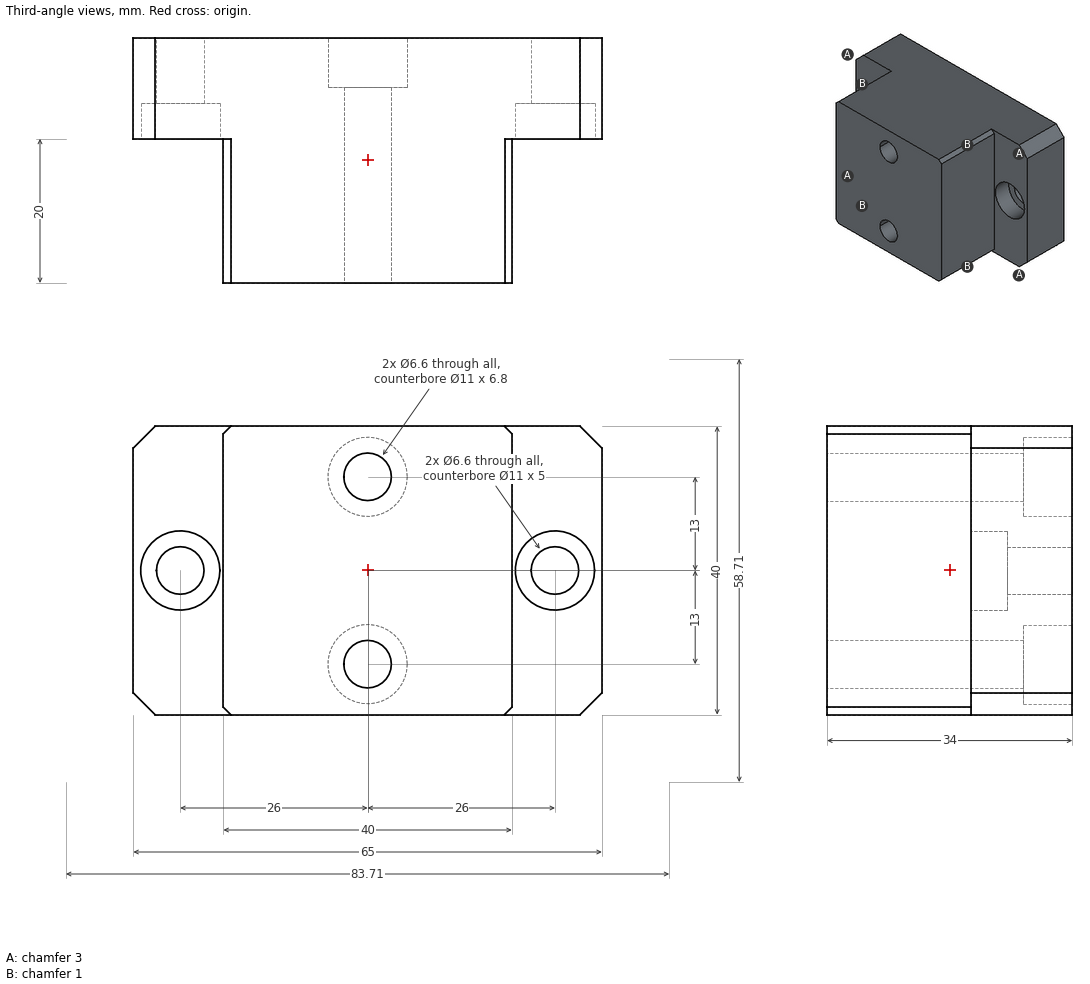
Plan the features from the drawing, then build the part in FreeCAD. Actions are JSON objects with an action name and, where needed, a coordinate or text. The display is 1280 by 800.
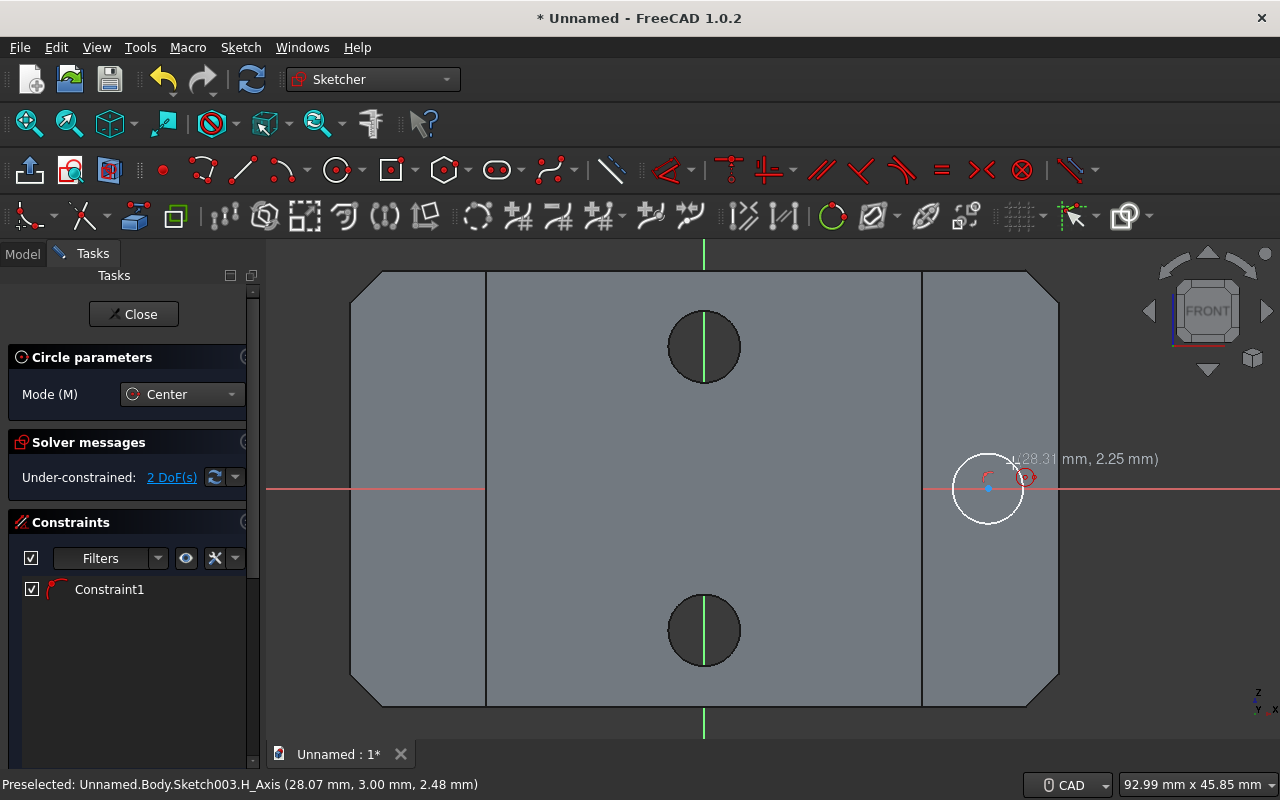
{"action": "left_click", "coordinate": [421, 489]}
{"action": "left_click", "coordinate": [446, 463]}
{"action": "key", "text": "Escape"}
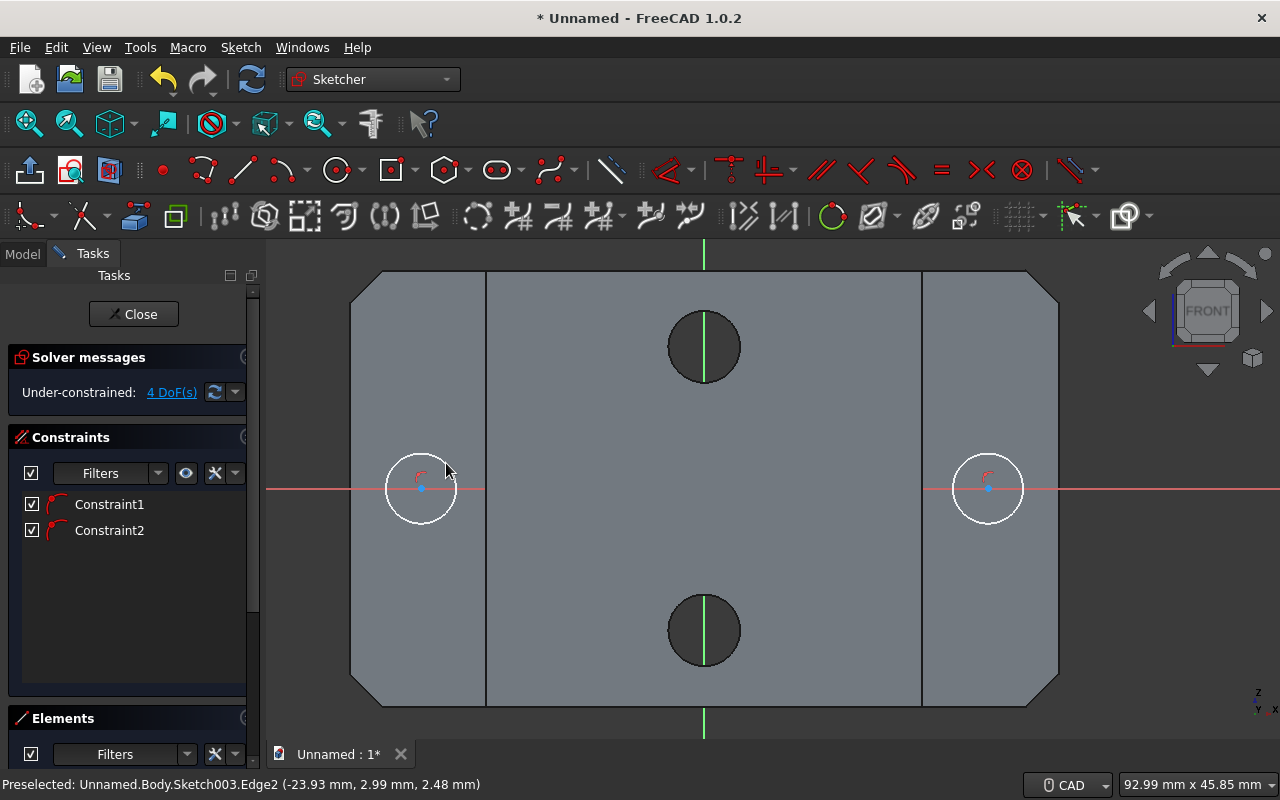
{"action": "left_click", "coordinate": [1013, 464]}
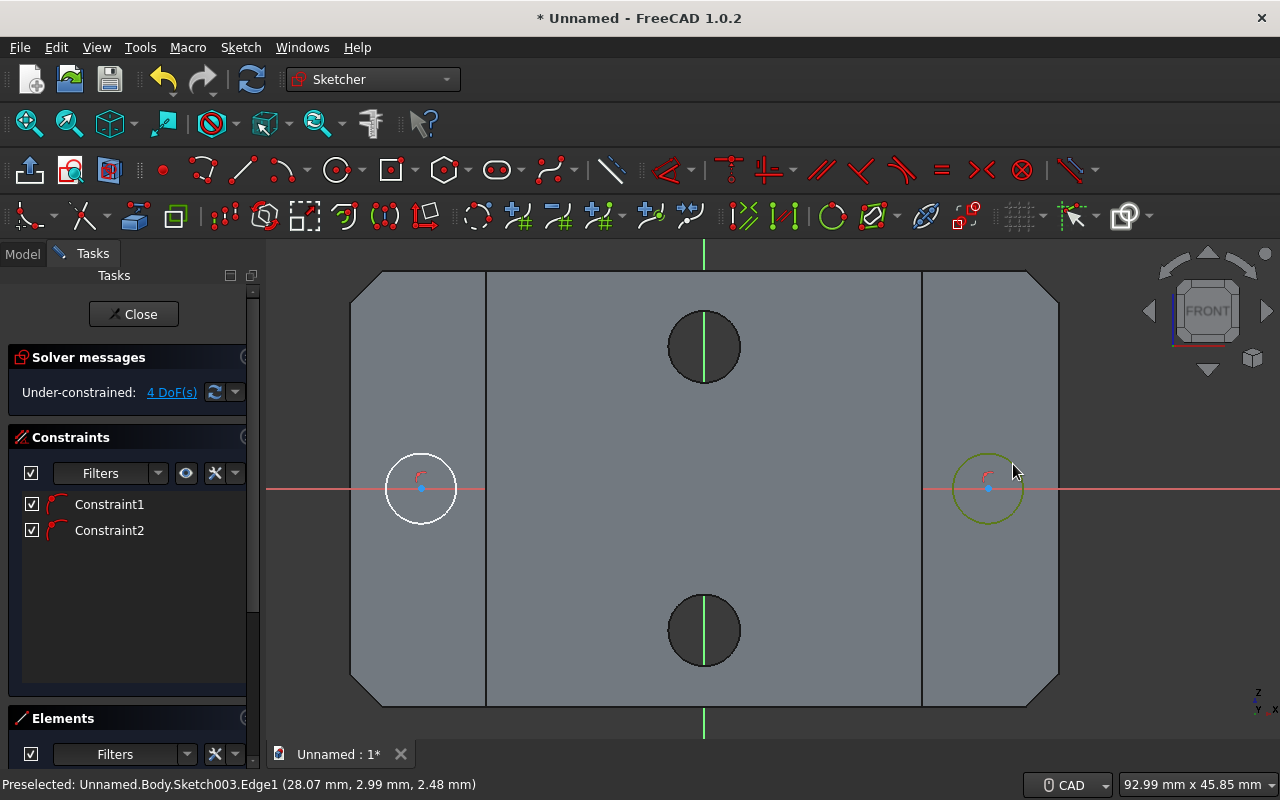
{"action": "left_click", "coordinate": [446, 464]}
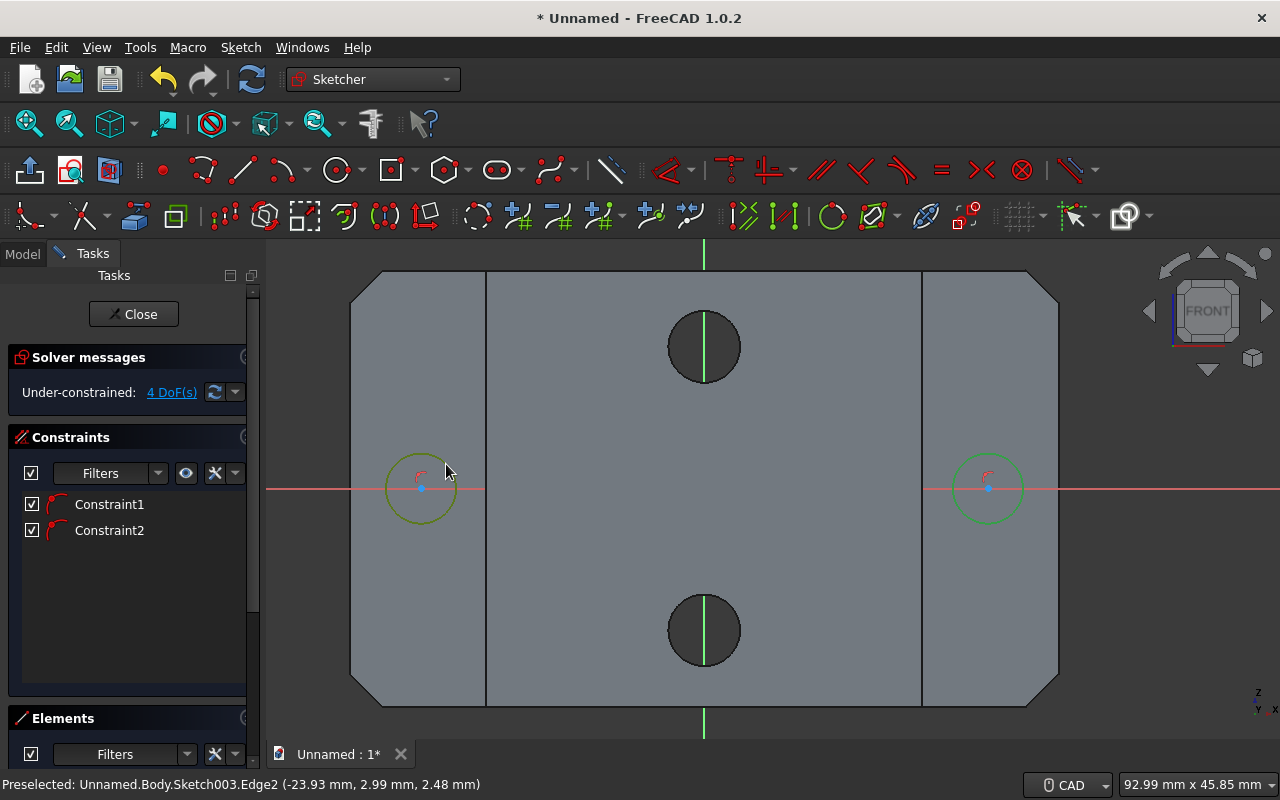
{"action": "key", "text": "e"}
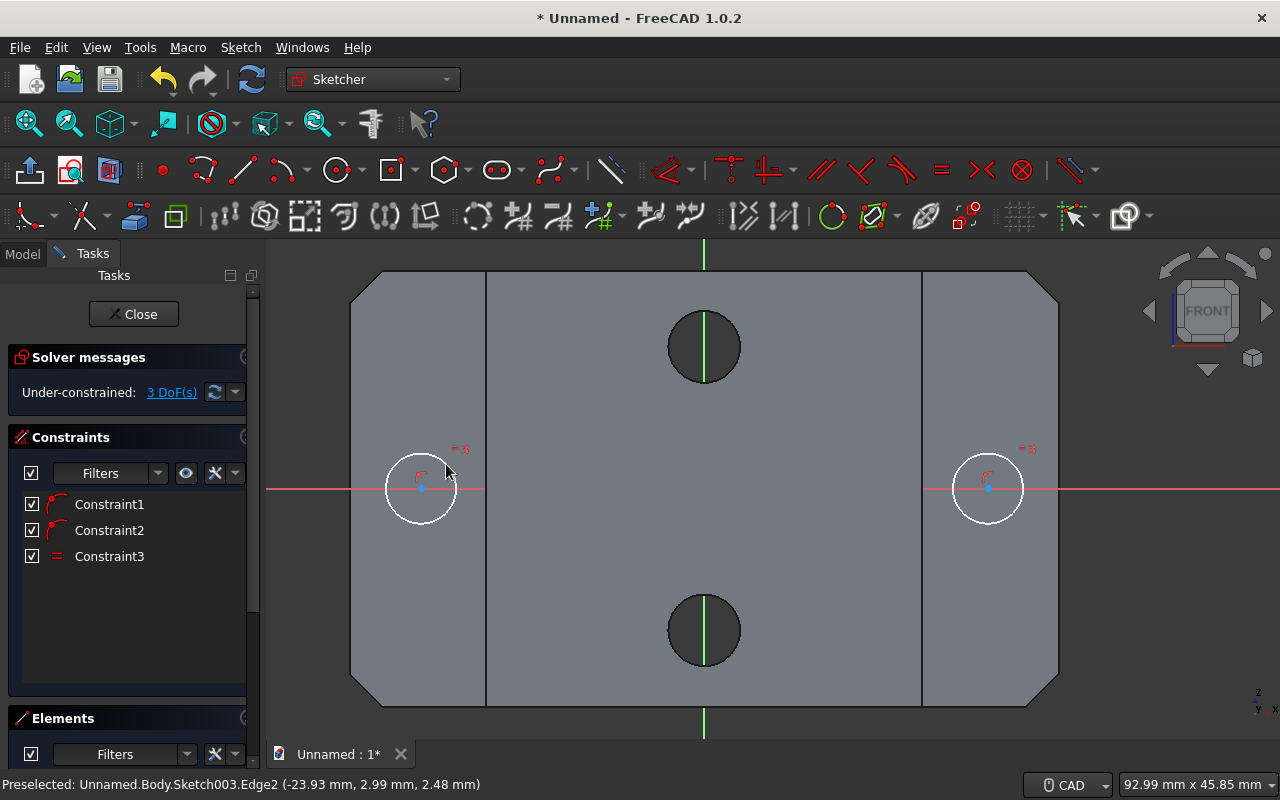
{"action": "key", "text": "d"}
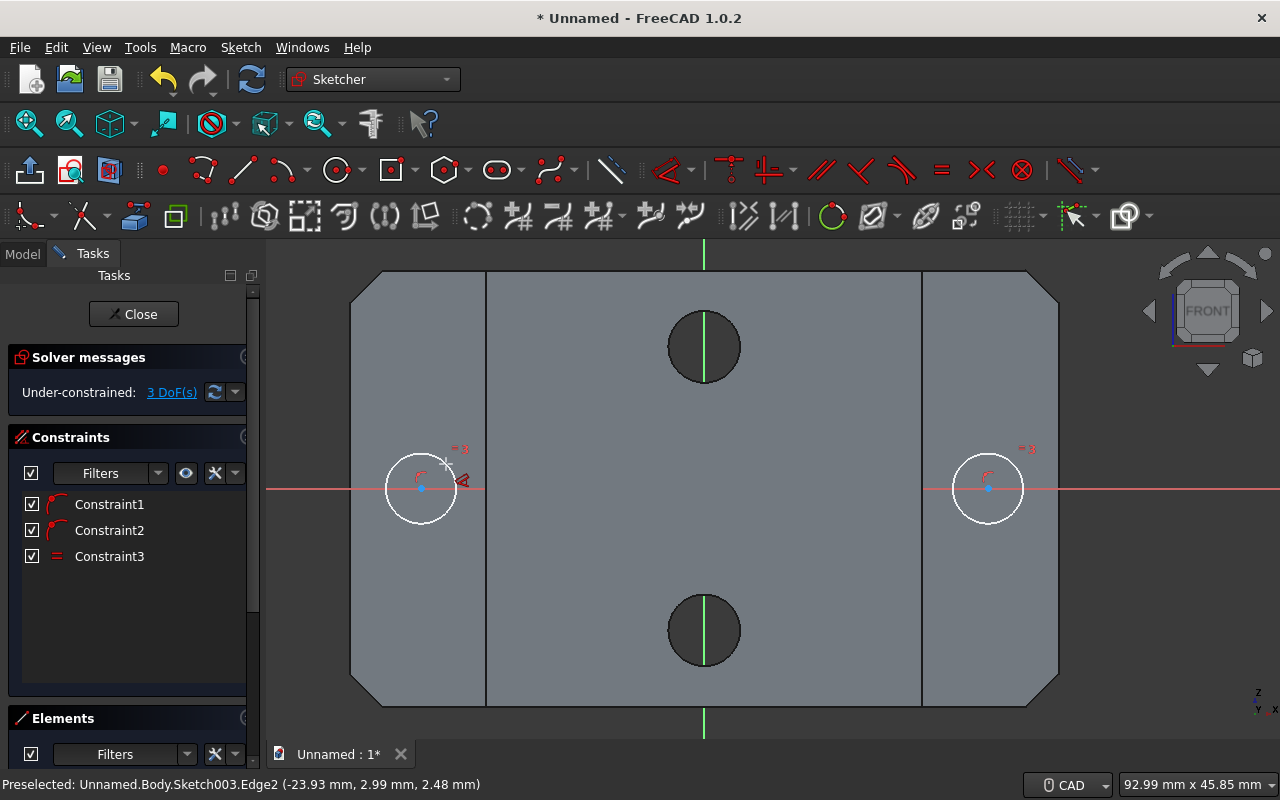
{"action": "left_click", "coordinate": [1013, 464]}
{"action": "left_click", "coordinate": [1036, 442]}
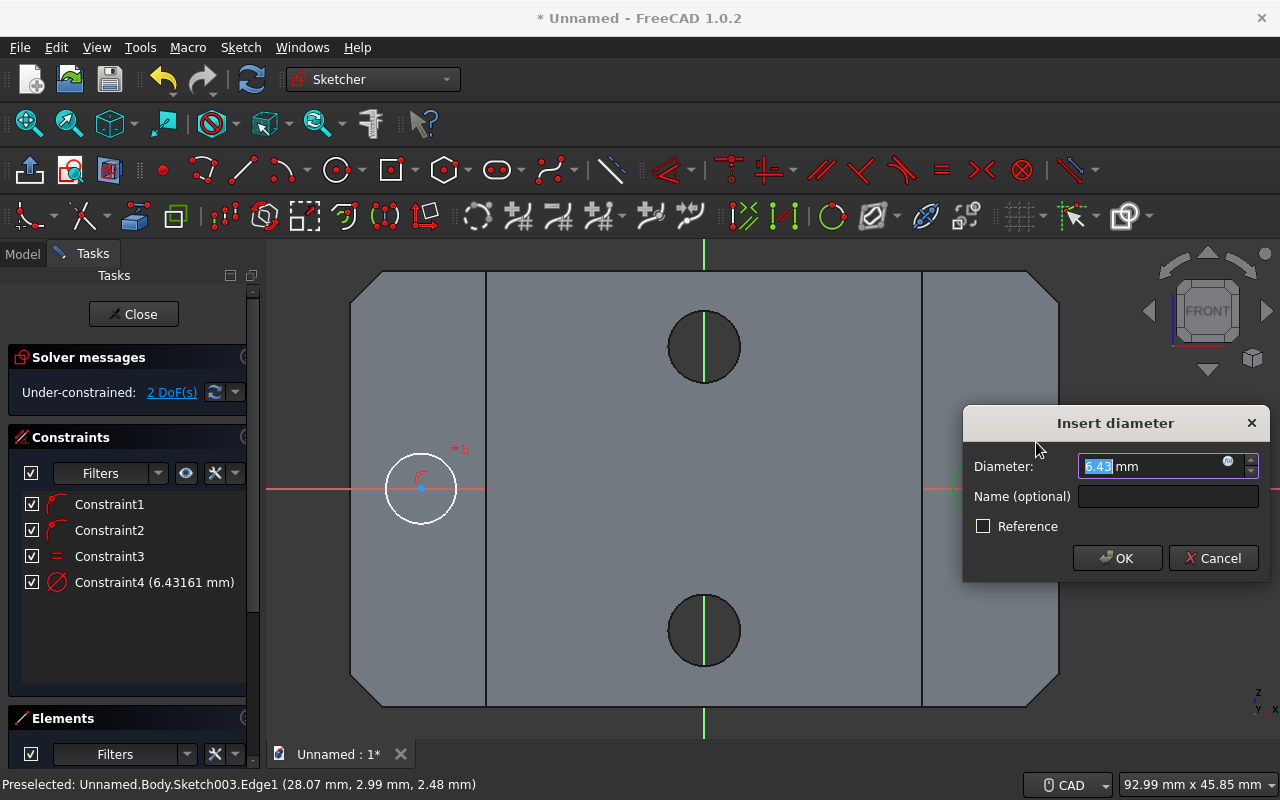
{"action": "type", "text": "6.6"}
{"action": "key", "text": "Return"}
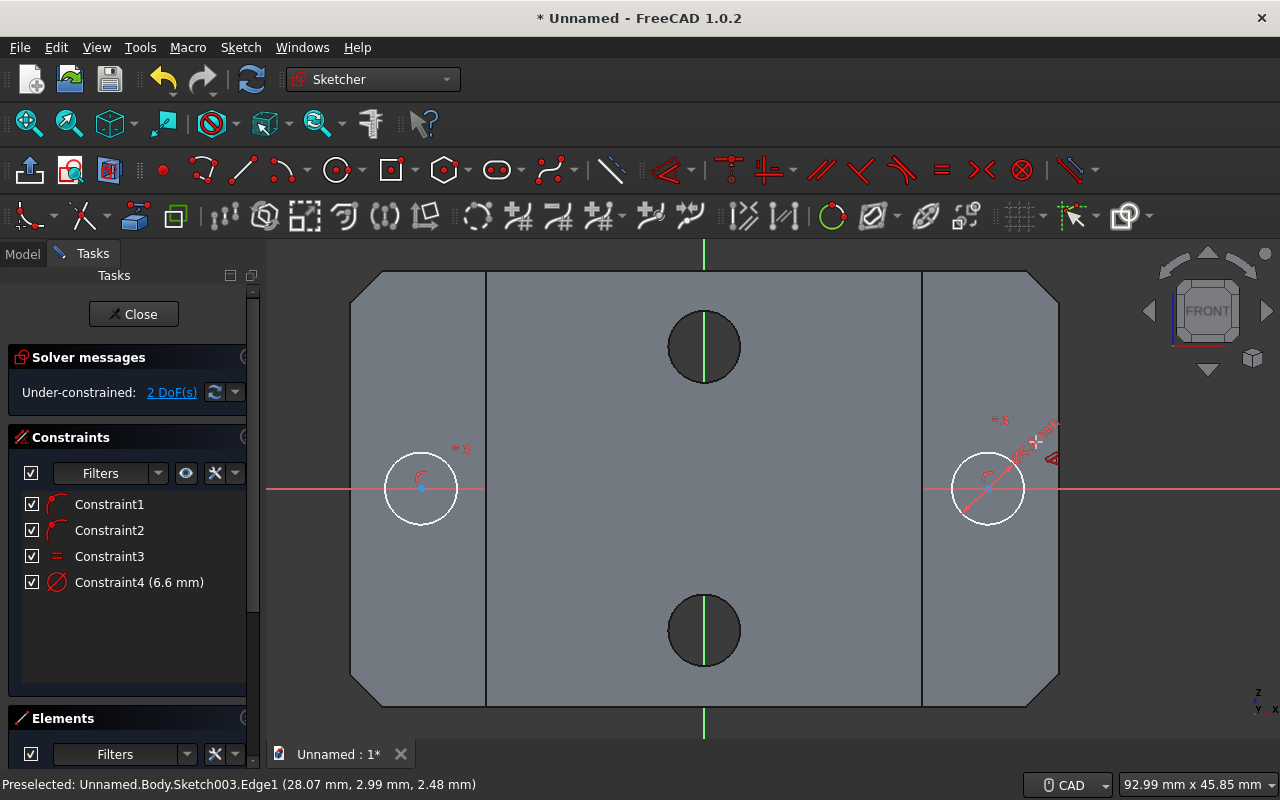
{"action": "left_click", "coordinate": [988, 489]}
{"action": "left_click", "coordinate": [846, 523]}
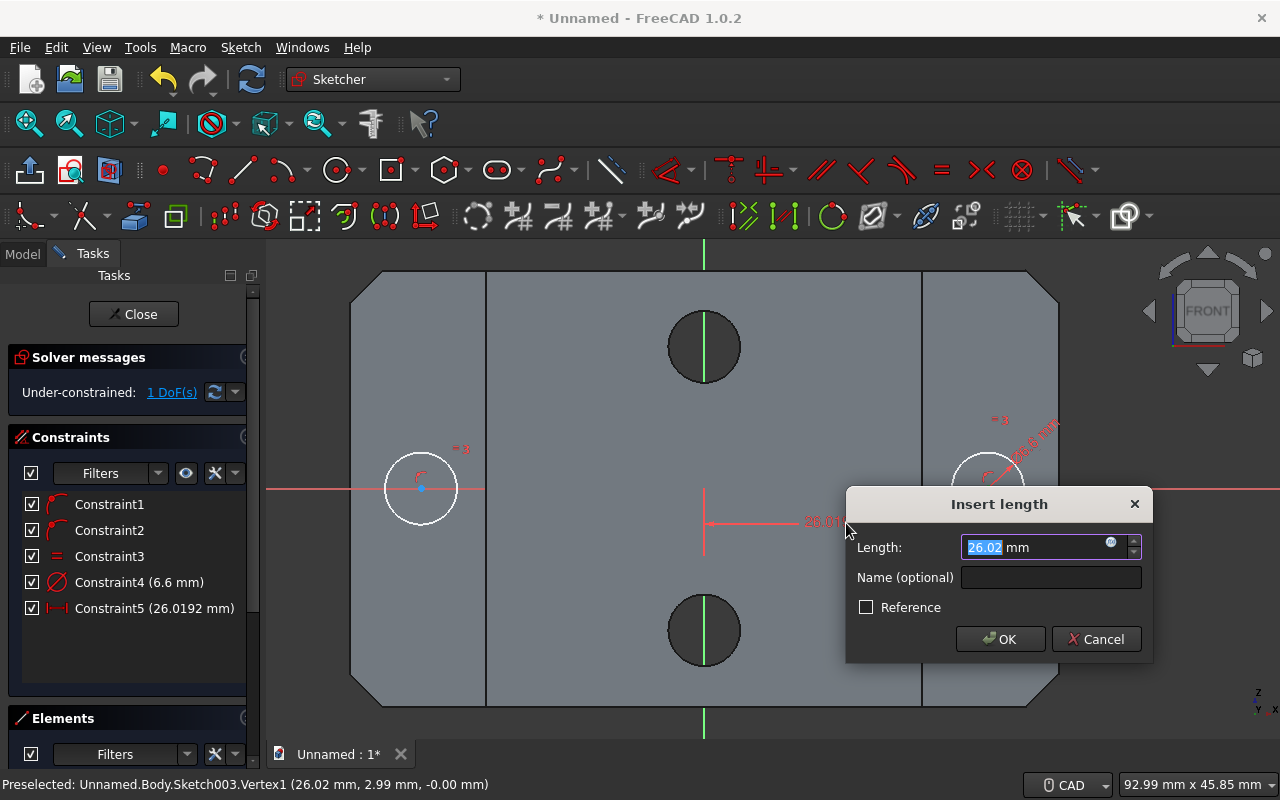
{"action": "type", "text": "26"}
{"action": "key", "text": "Return"}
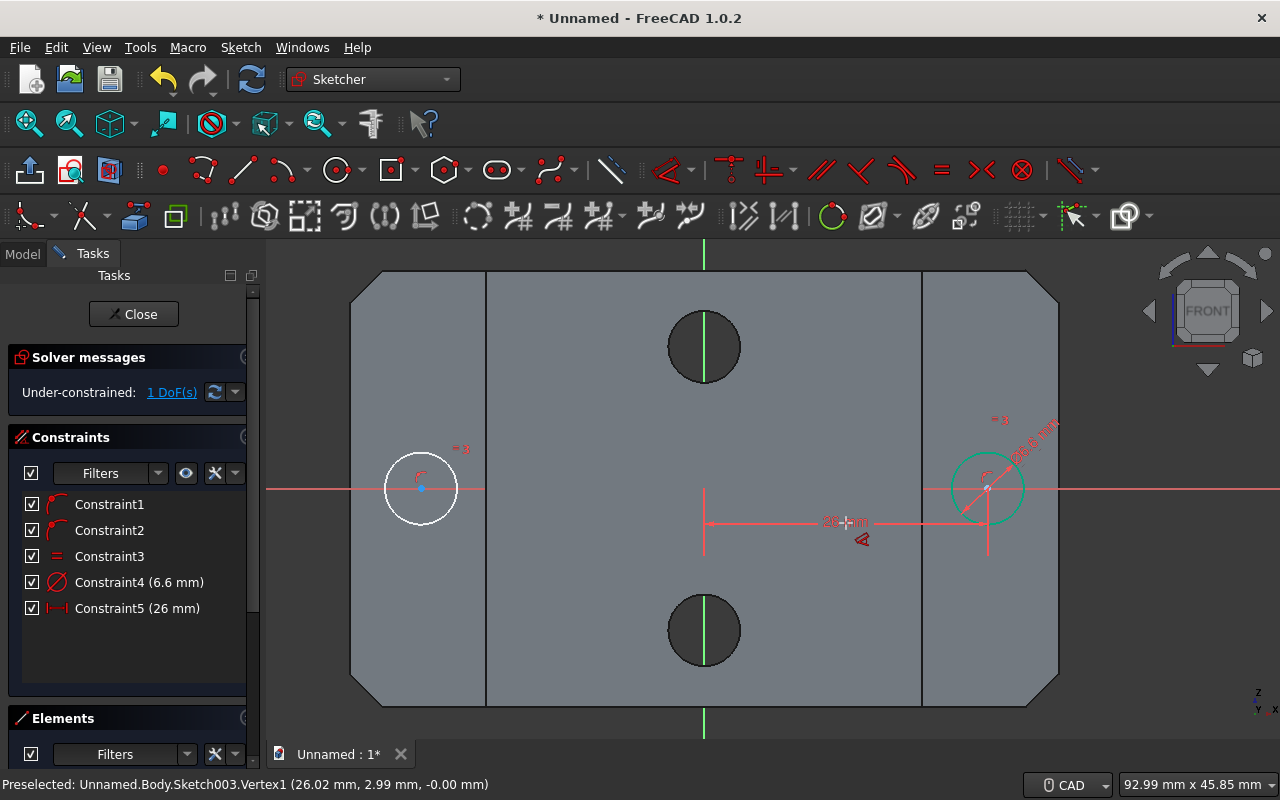
{"action": "left_click", "coordinate": [421, 489]}
{"action": "left_click", "coordinate": [563, 523]}